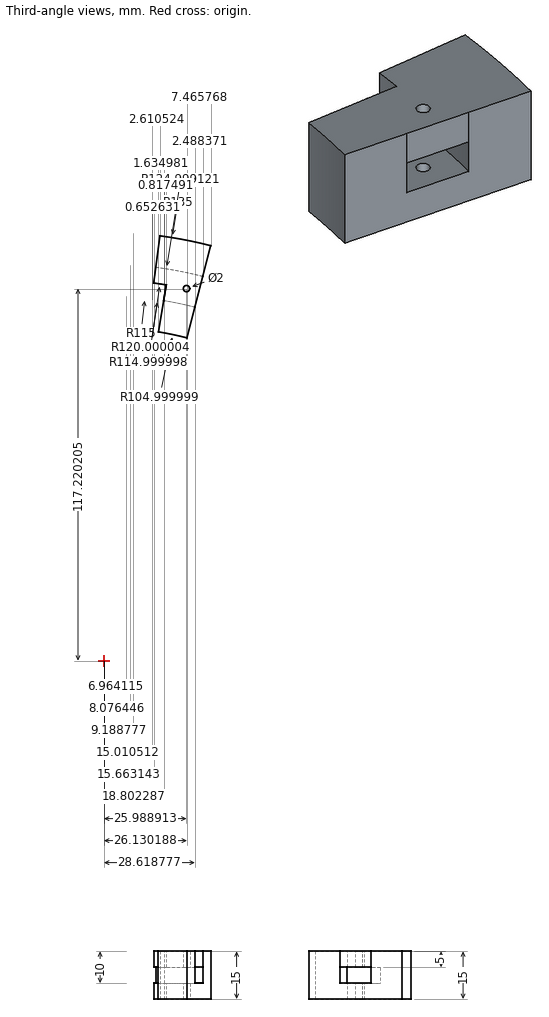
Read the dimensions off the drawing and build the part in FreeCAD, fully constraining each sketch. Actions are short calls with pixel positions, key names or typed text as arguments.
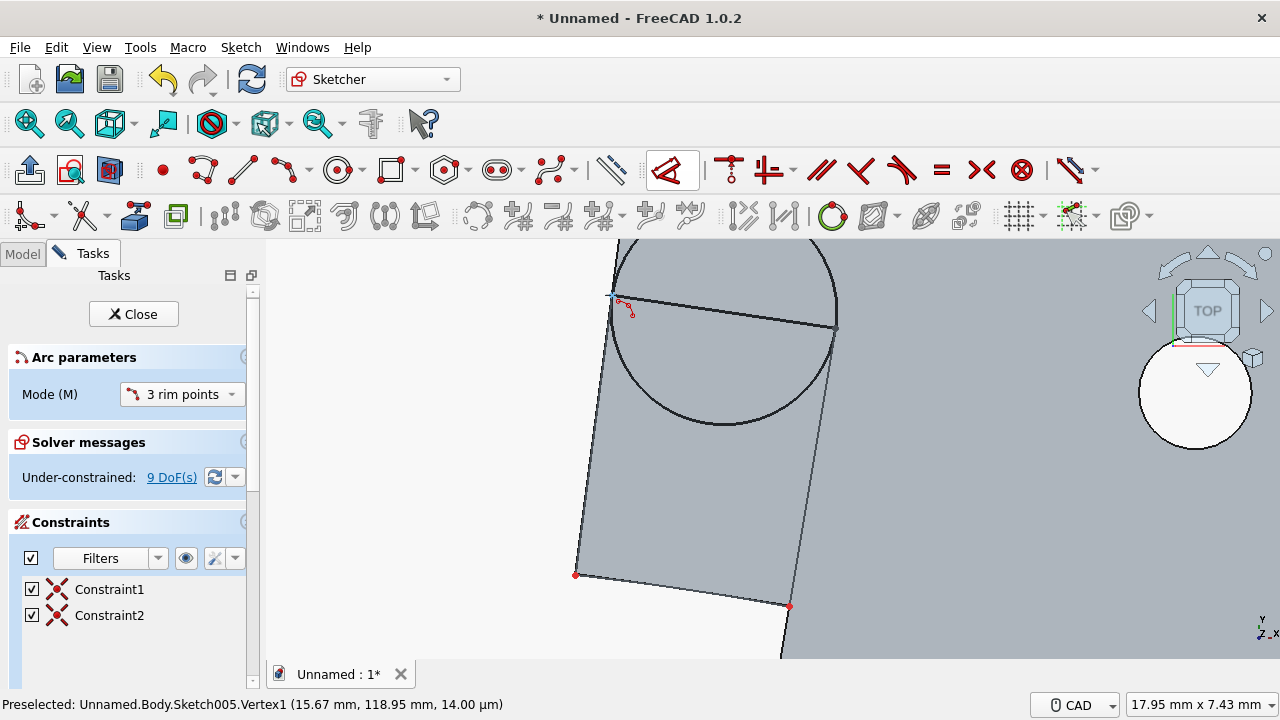
scroll(724, 309, up, 15)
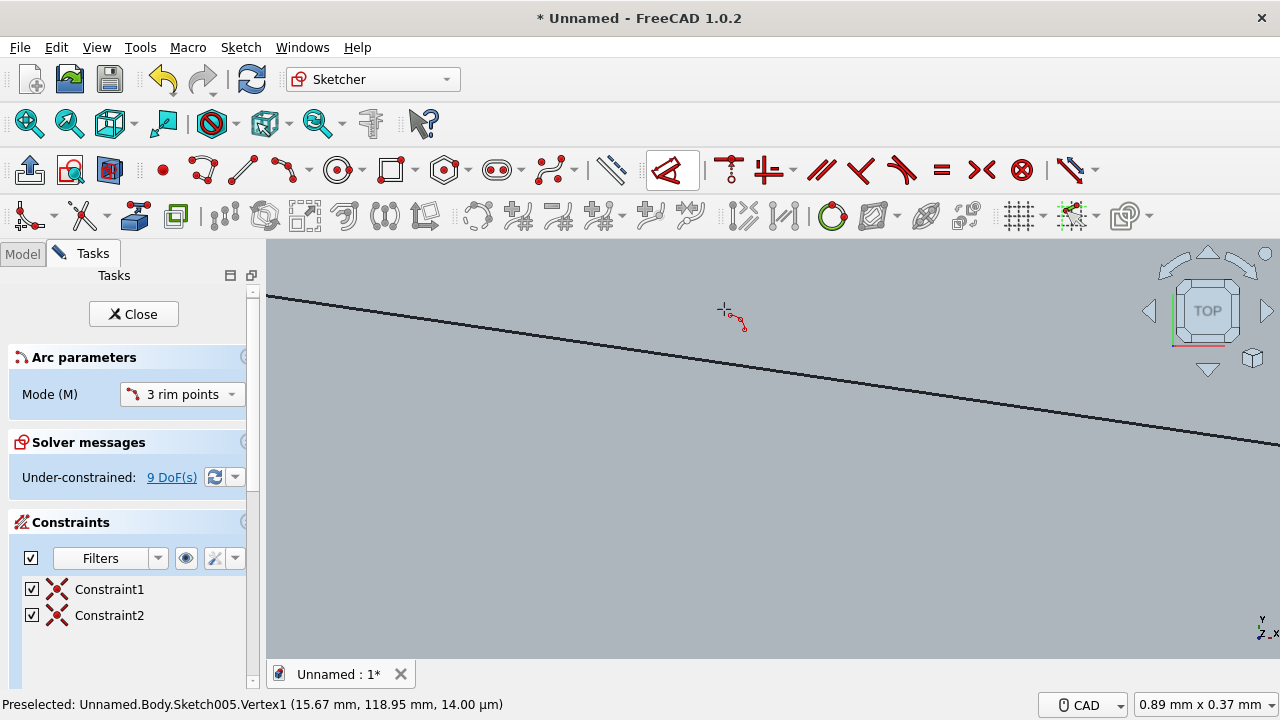
click(713, 315)
key(Escape)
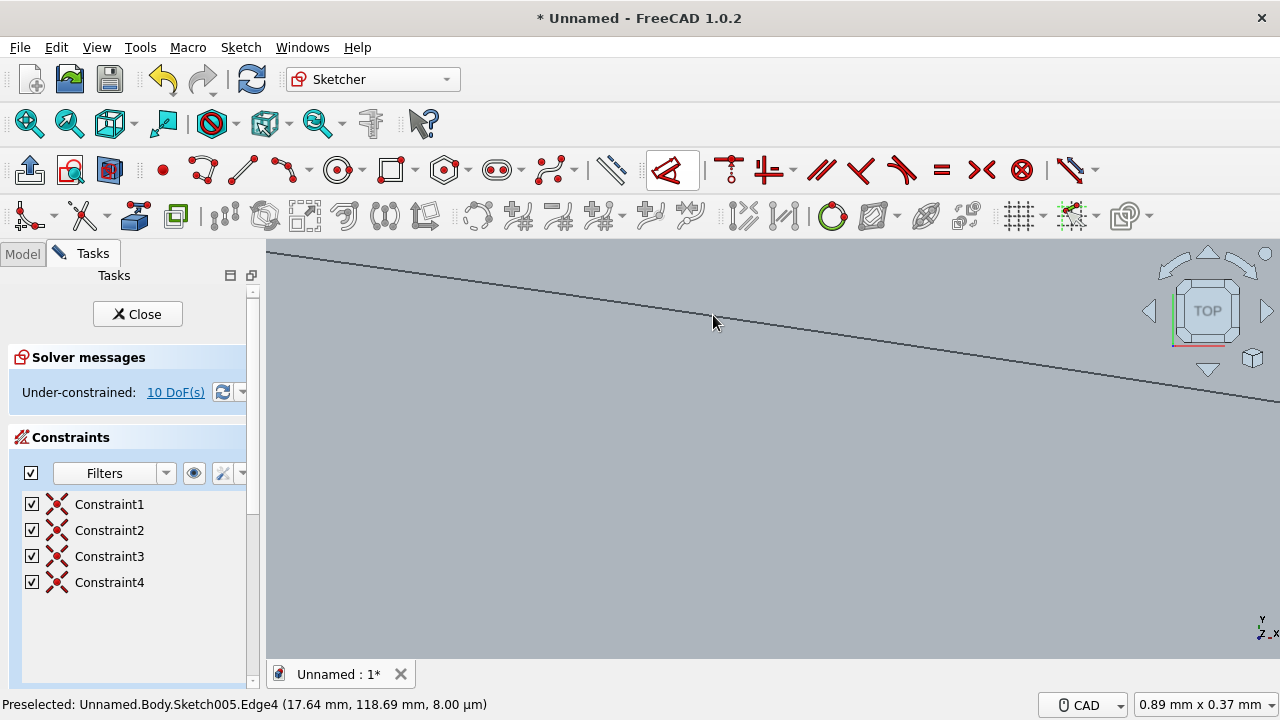
scroll(724, 308, down, 15)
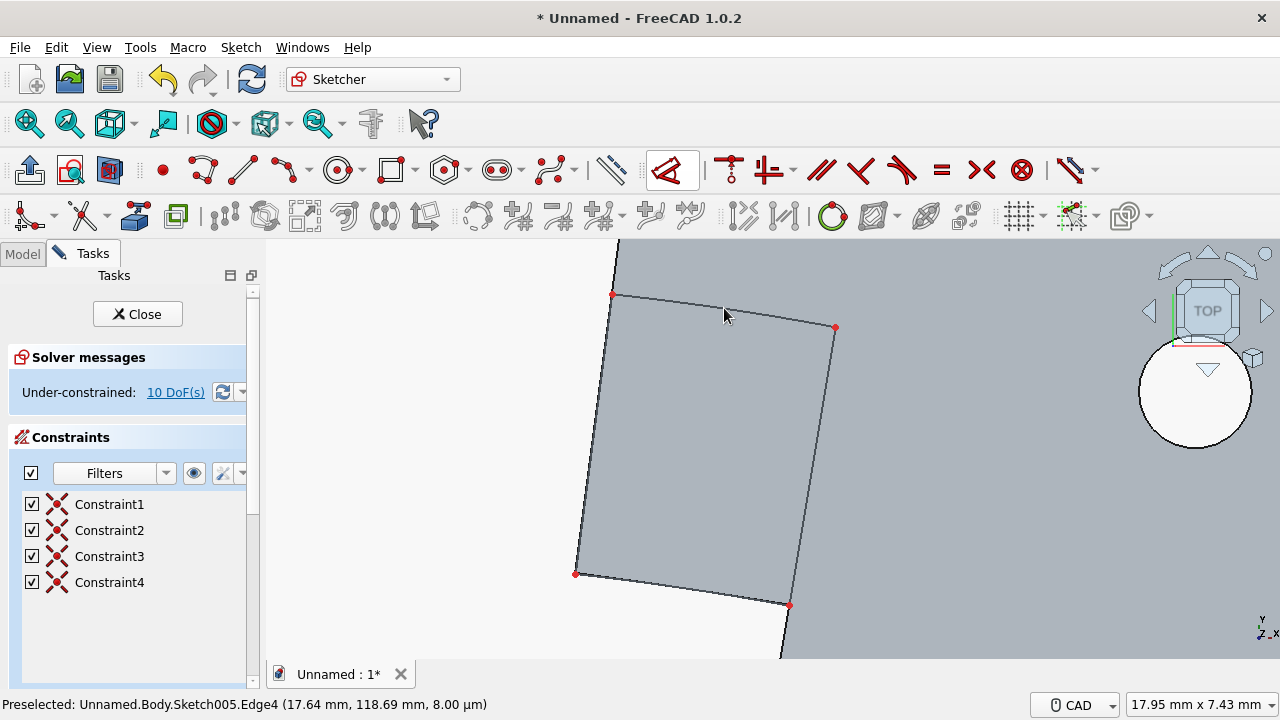
click(726, 595)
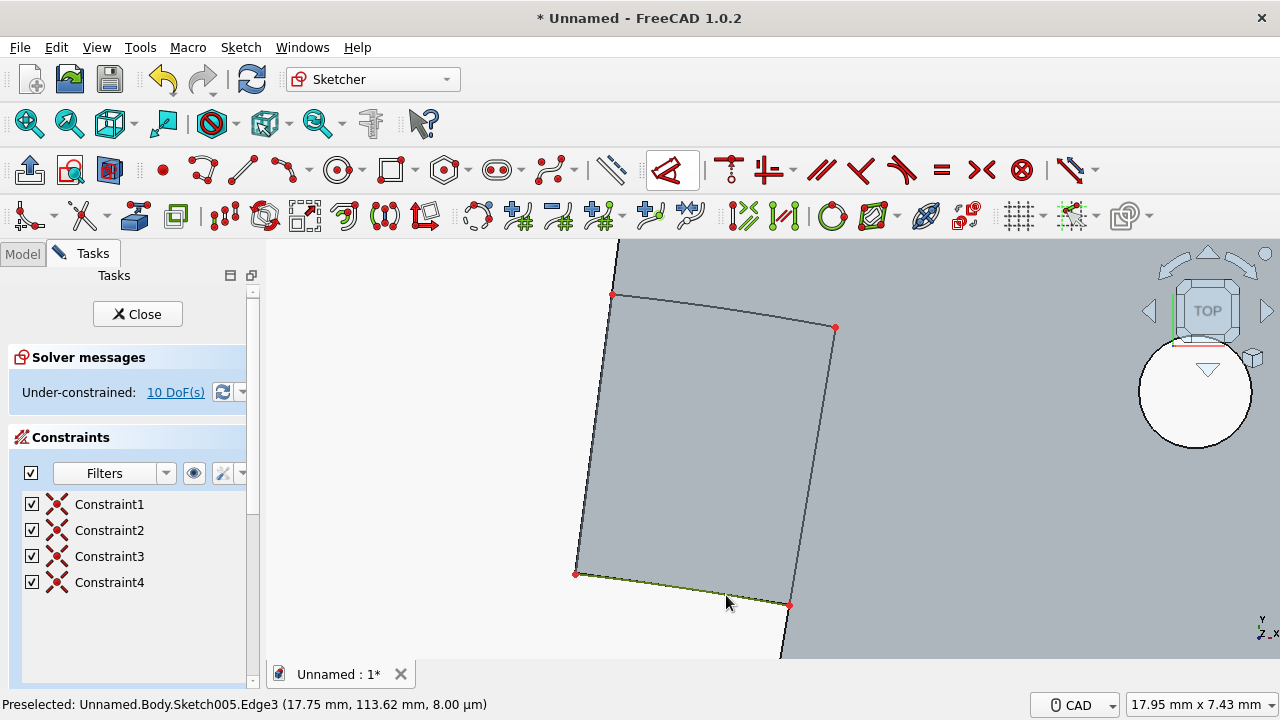
click(769, 316)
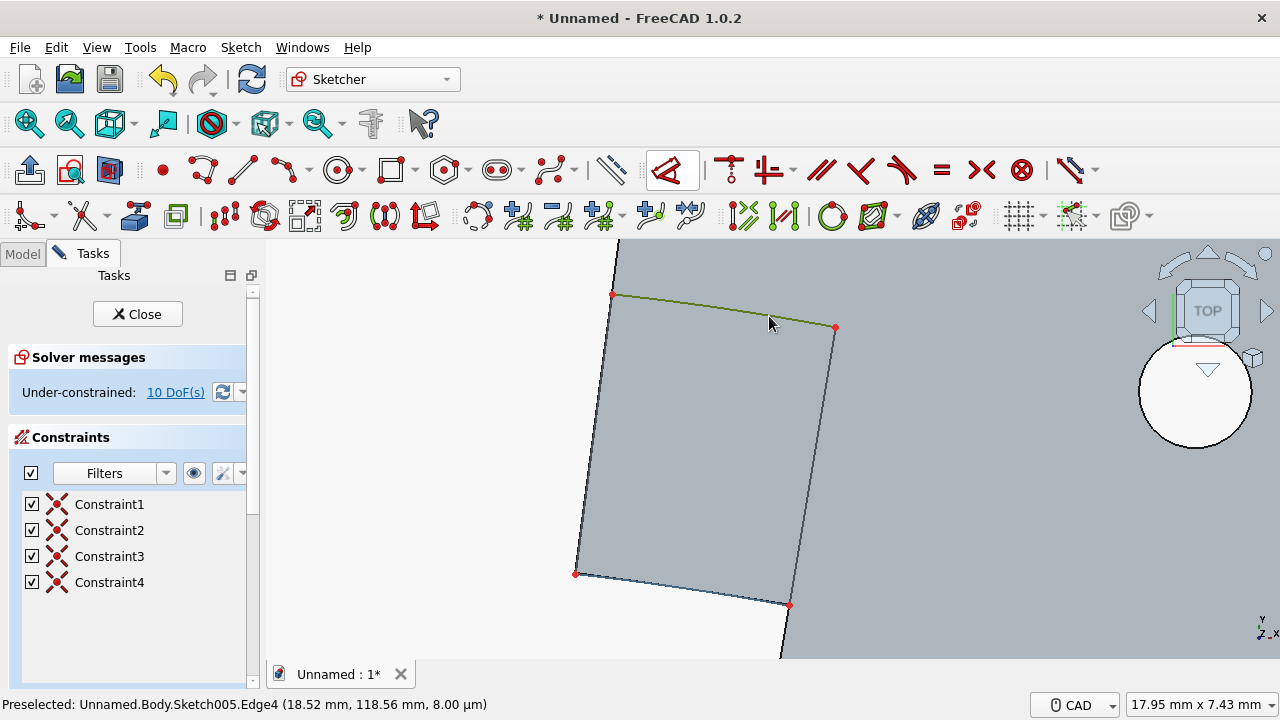
click(730, 170)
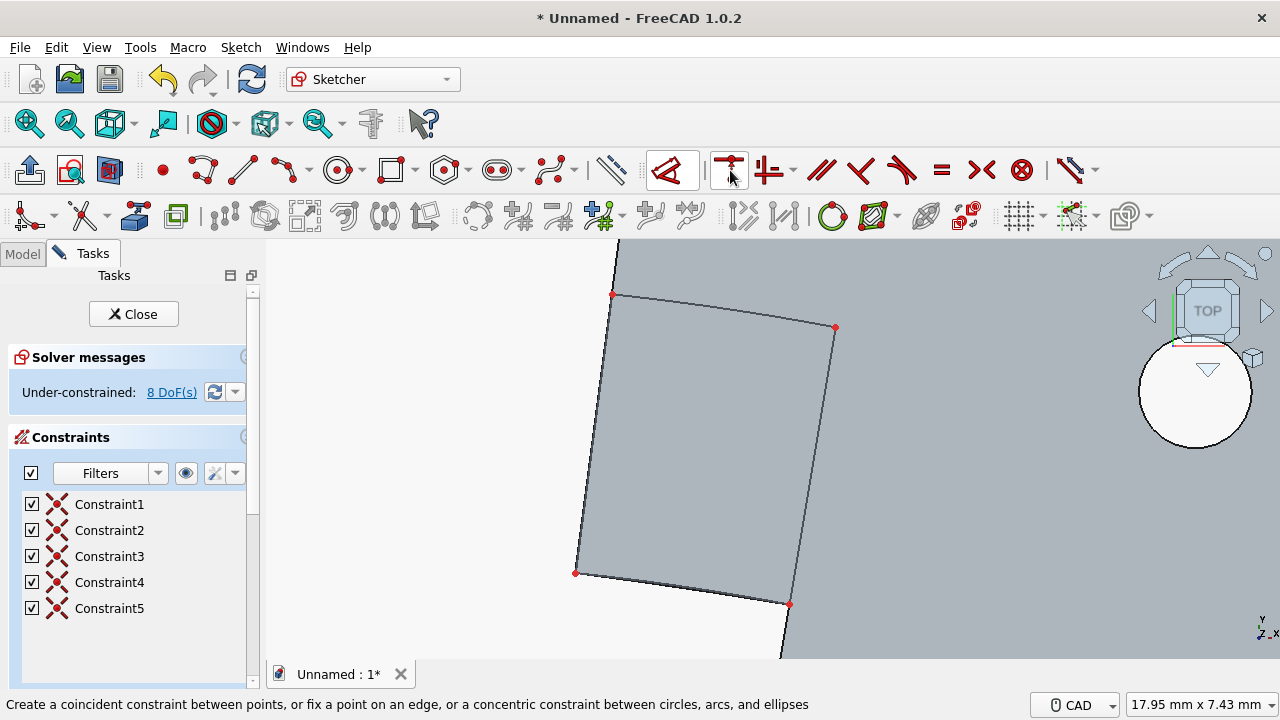
scroll(719, 332, down, 15)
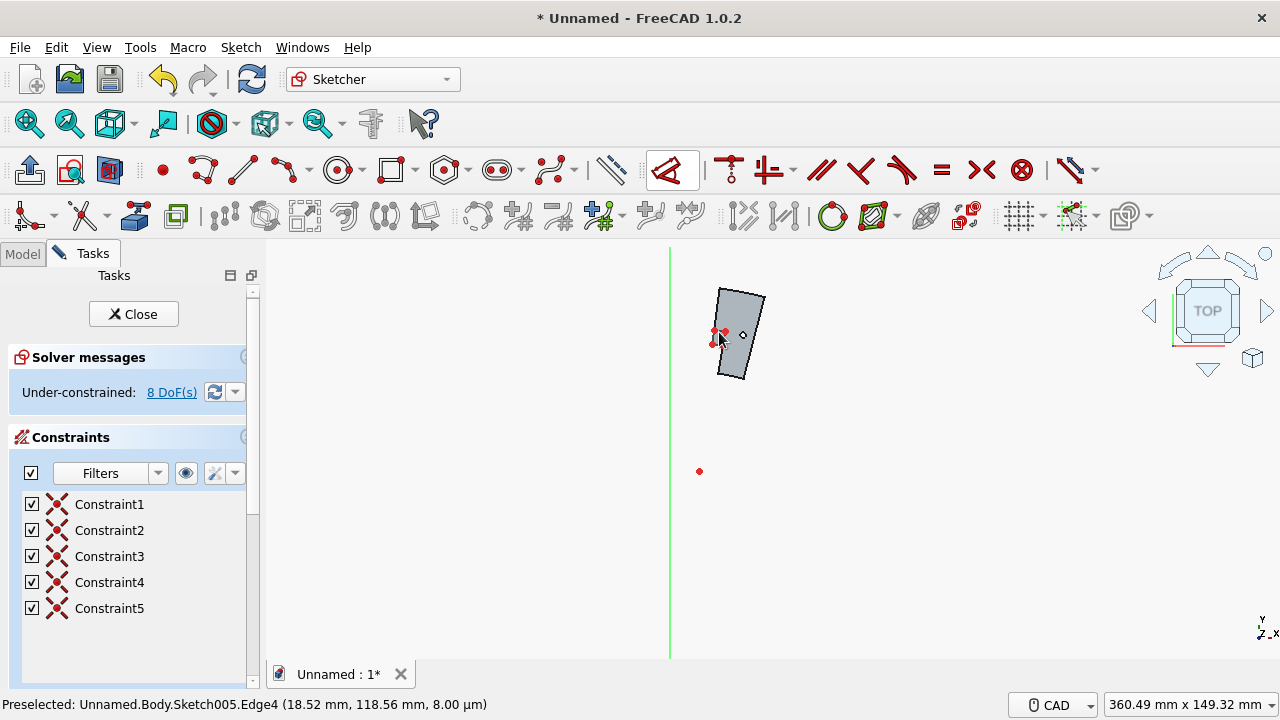
drag(660, 461, 709, 675)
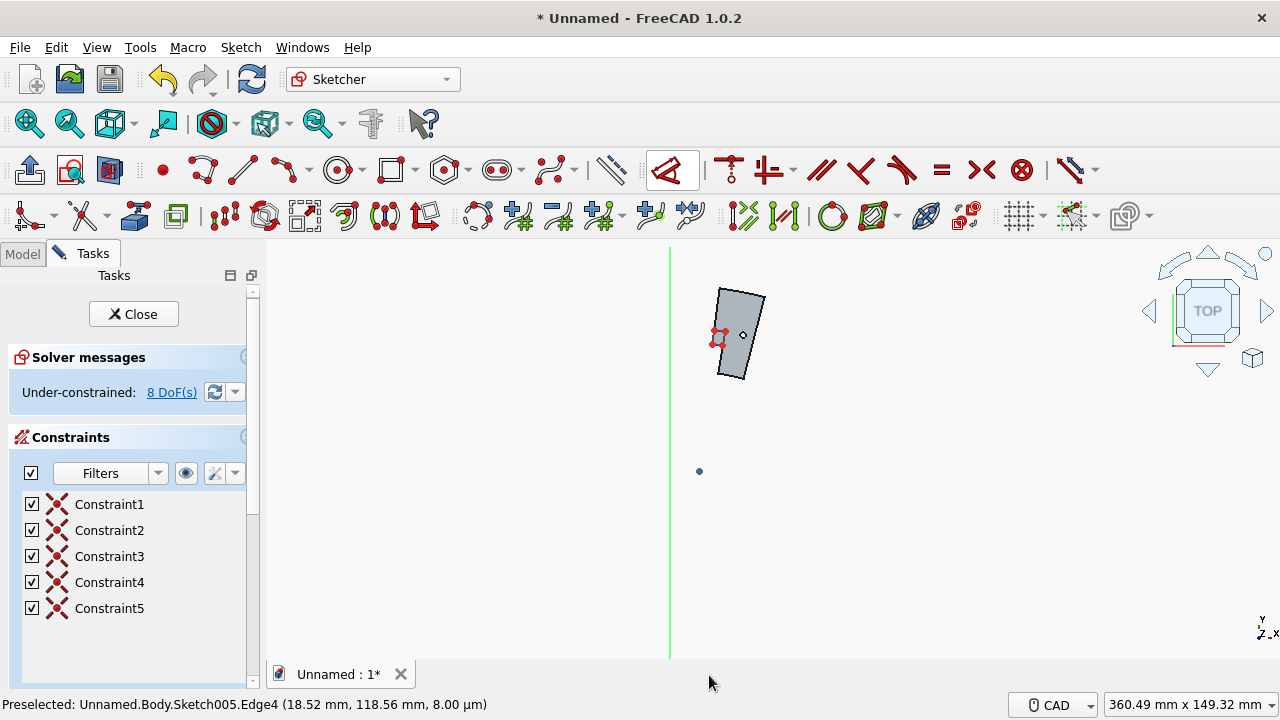
click(730, 170)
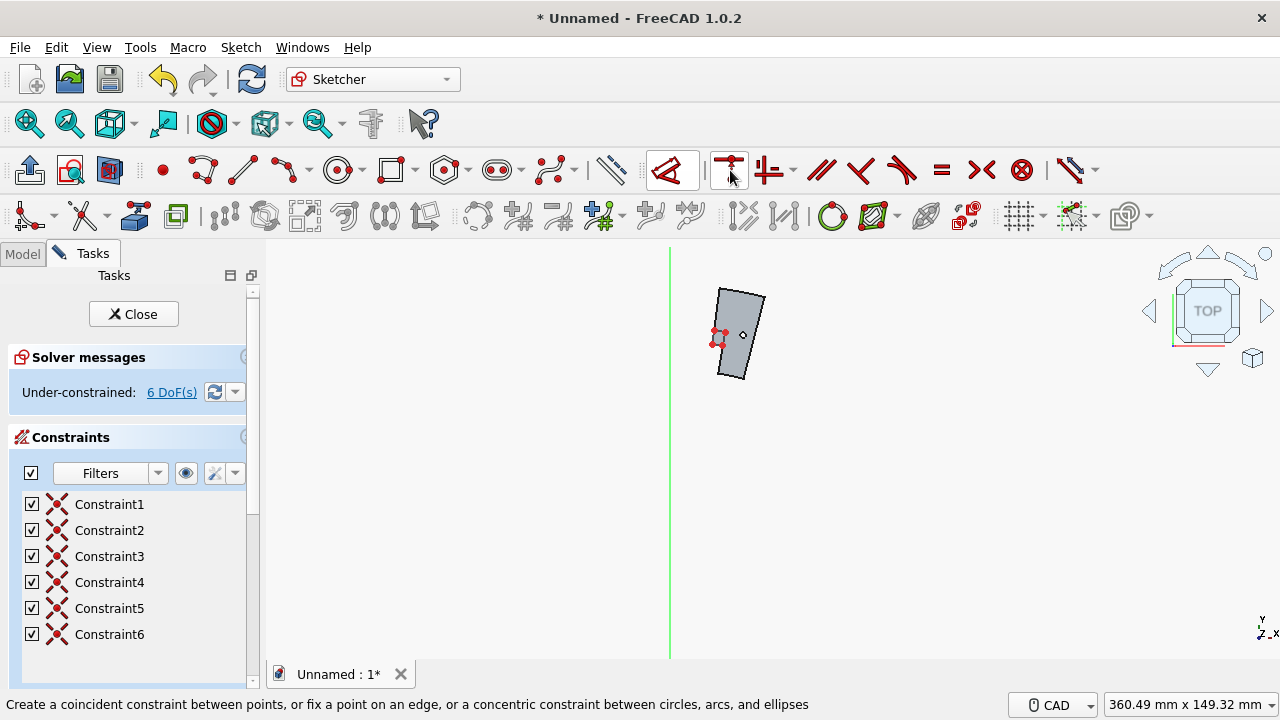
scroll(718, 345, up, 5)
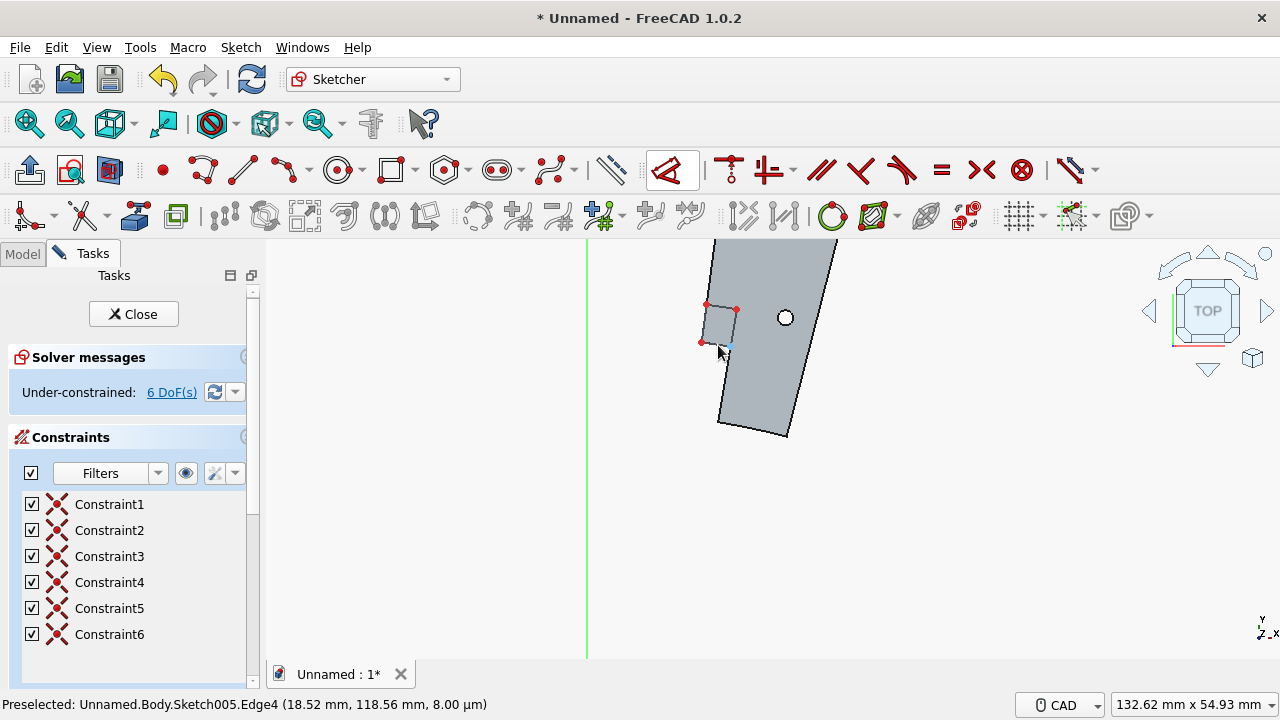
click(716, 344)